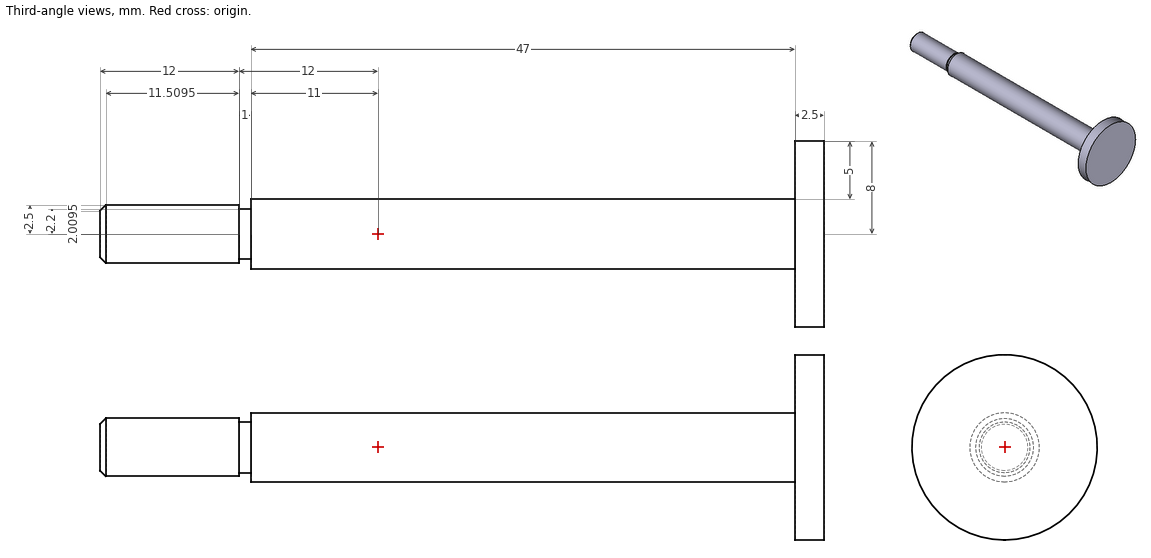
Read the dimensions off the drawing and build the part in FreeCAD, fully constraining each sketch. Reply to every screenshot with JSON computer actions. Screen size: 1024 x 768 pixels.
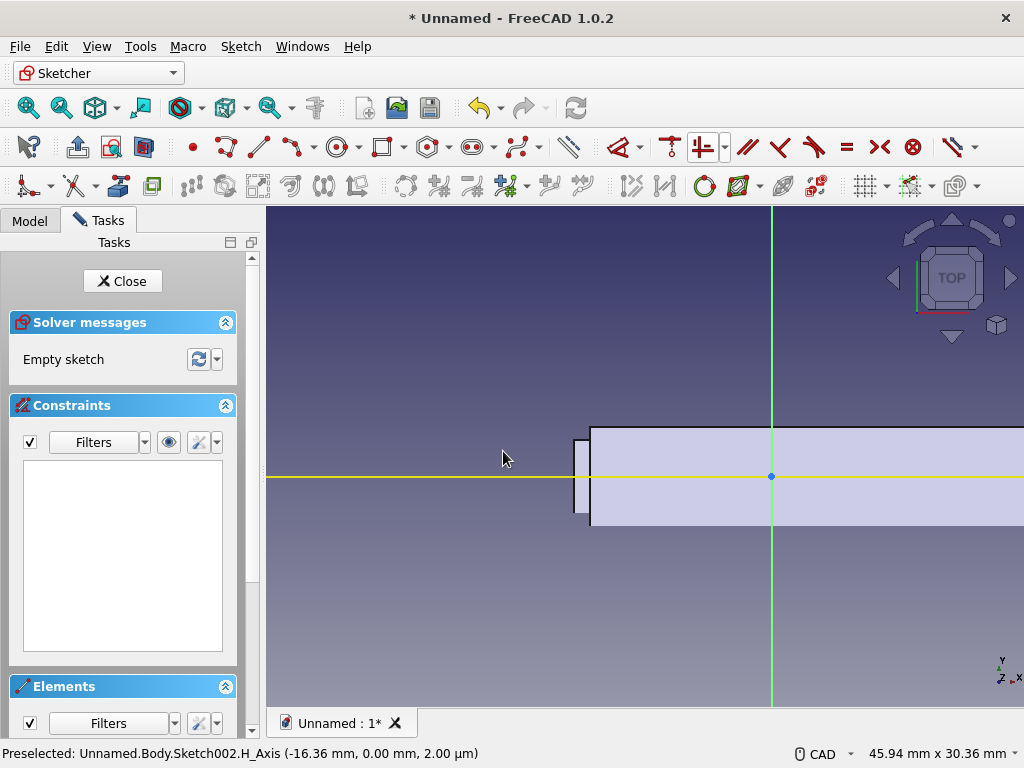
{"action": "key", "text": "g m"}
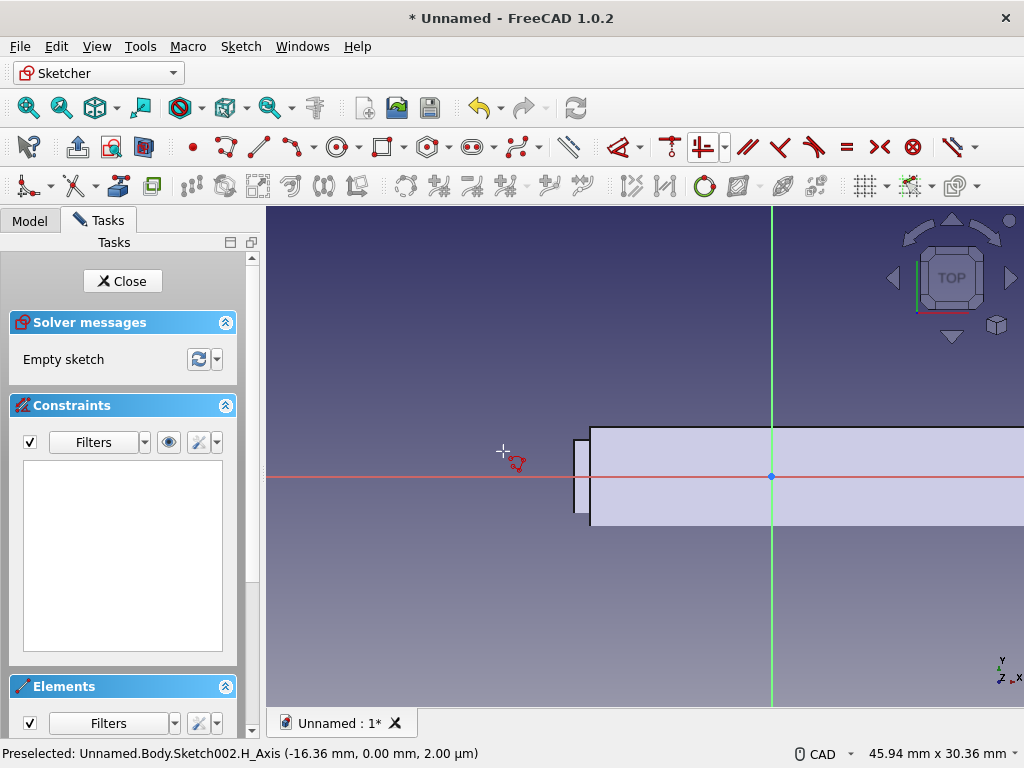
{"action": "left_click", "coordinate": [574, 477]}
{"action": "left_click", "coordinate": [574, 435]}
{"action": "left_click", "coordinate": [384, 435]}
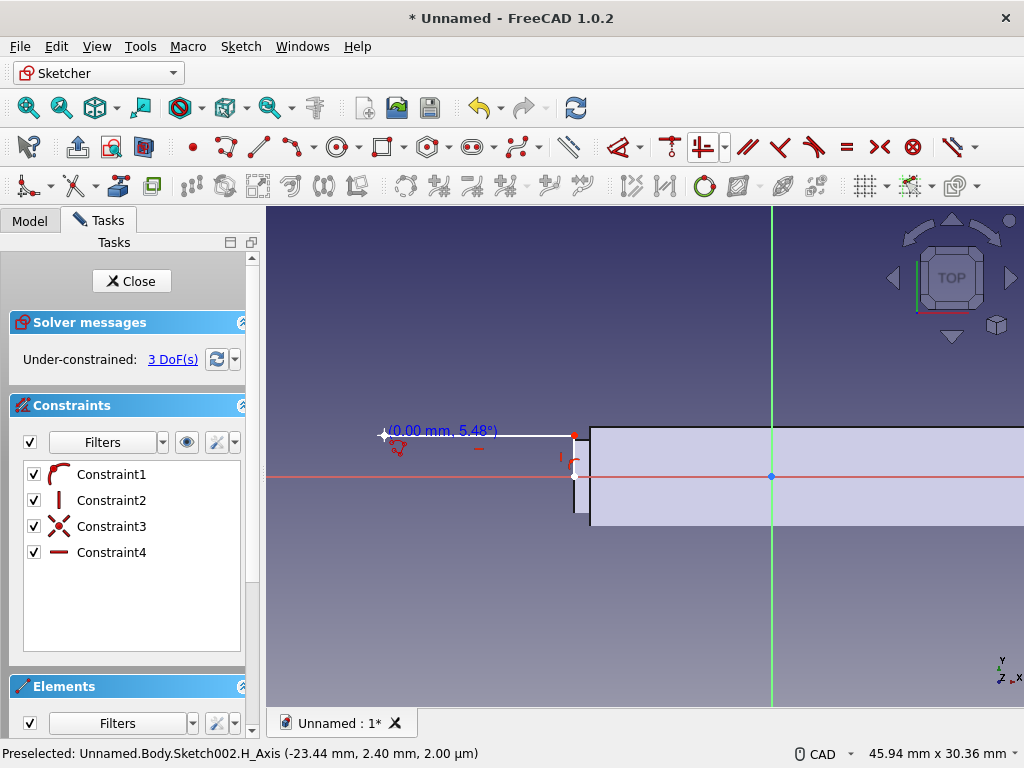
{"action": "scroll", "coordinate": [376, 443], "scroll_direction": "up", "scroll_amount": 2}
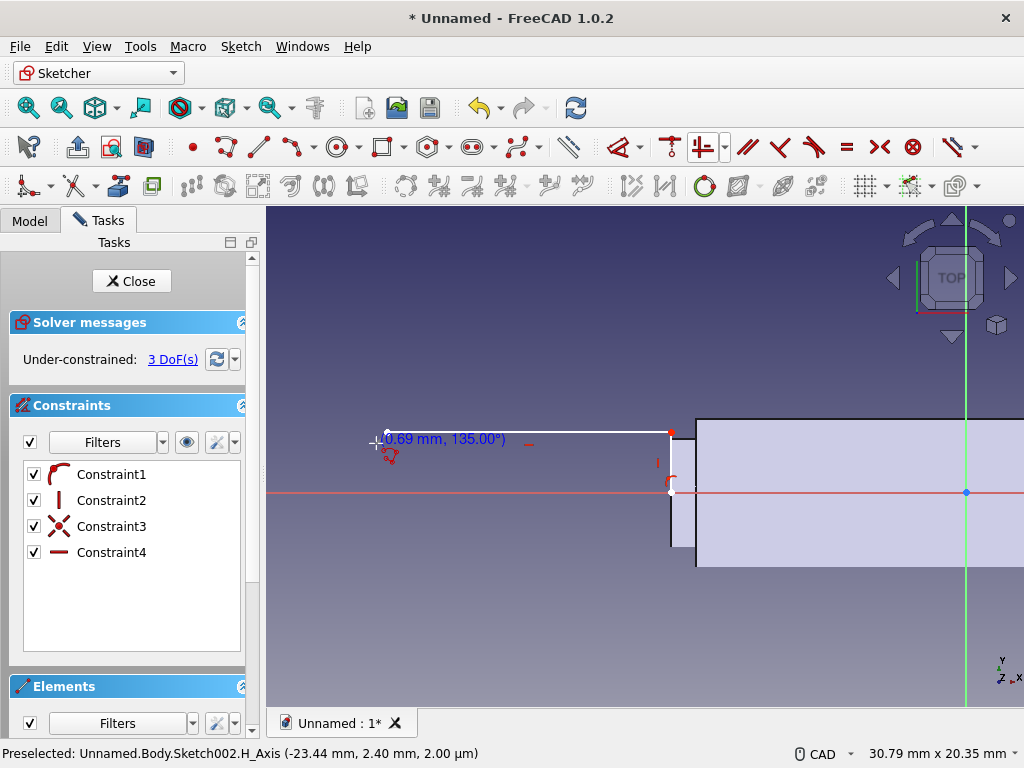
{"action": "left_click", "coordinate": [376, 443]}
{"action": "left_click", "coordinate": [376, 484]}
{"action": "left_click", "coordinate": [671, 493]}
{"action": "key", "text": "Escape"}
{"action": "key", "text": "Escape"}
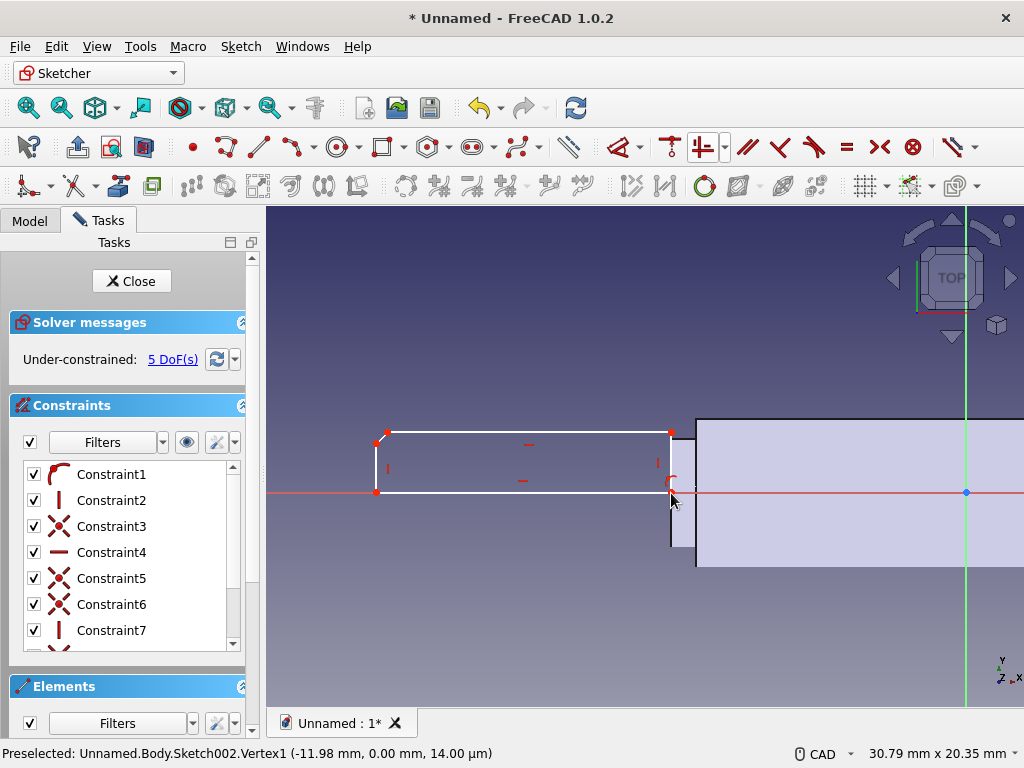
{"action": "left_click", "coordinate": [618, 148]}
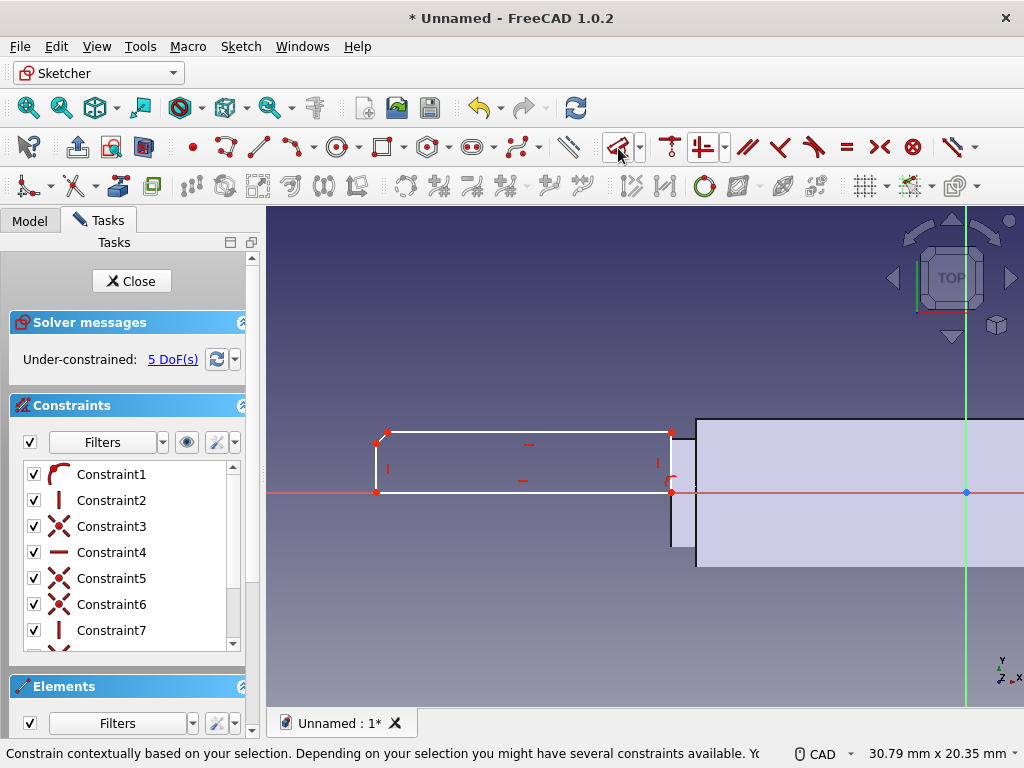
{"action": "left_click", "coordinate": [465, 493]}
{"action": "left_click", "coordinate": [524, 527]}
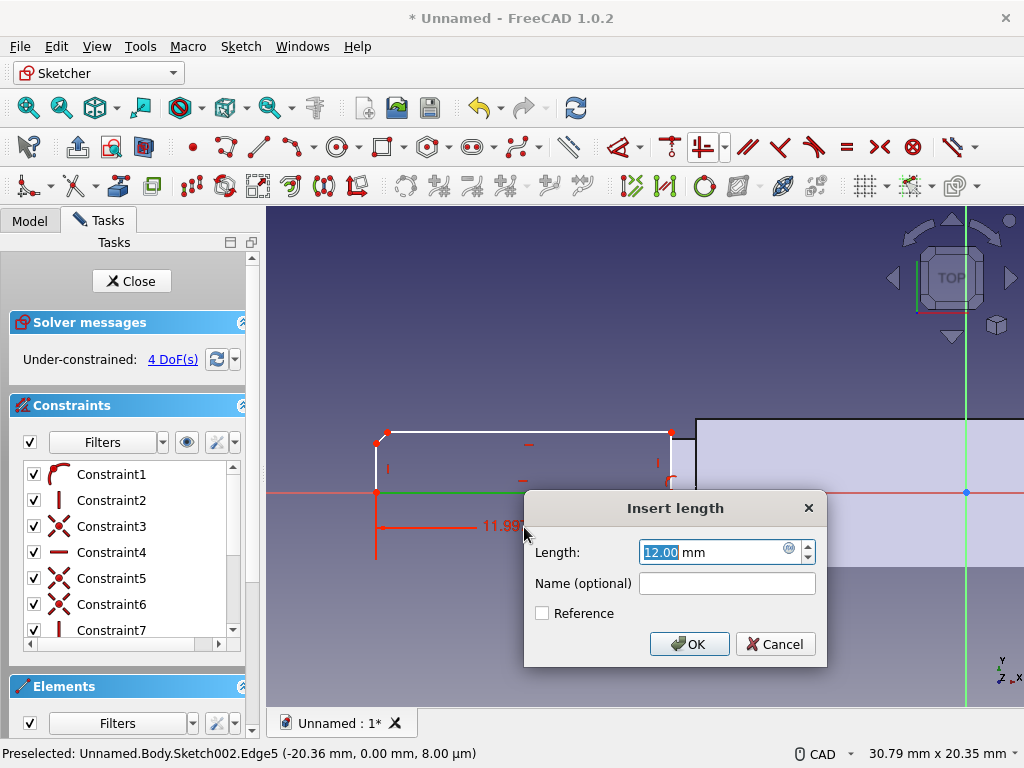
{"action": "type", "text": "12"}
{"action": "key", "text": "Return"}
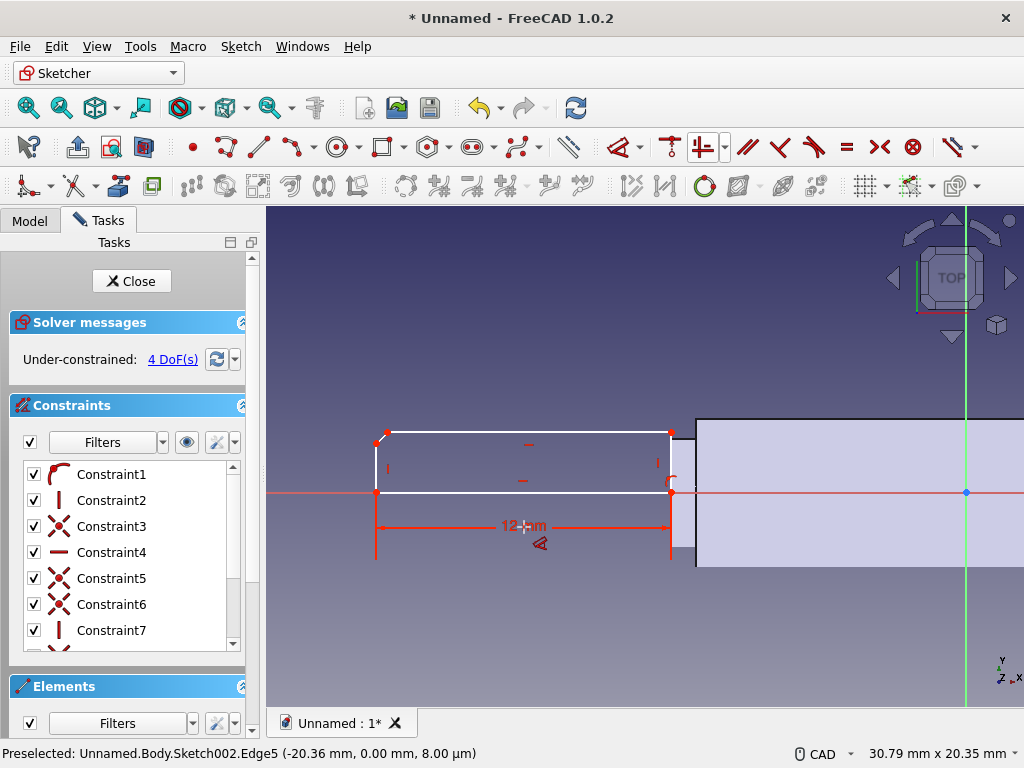
{"action": "left_click", "coordinate": [671, 475]}
{"action": "left_click", "coordinate": [705, 463]}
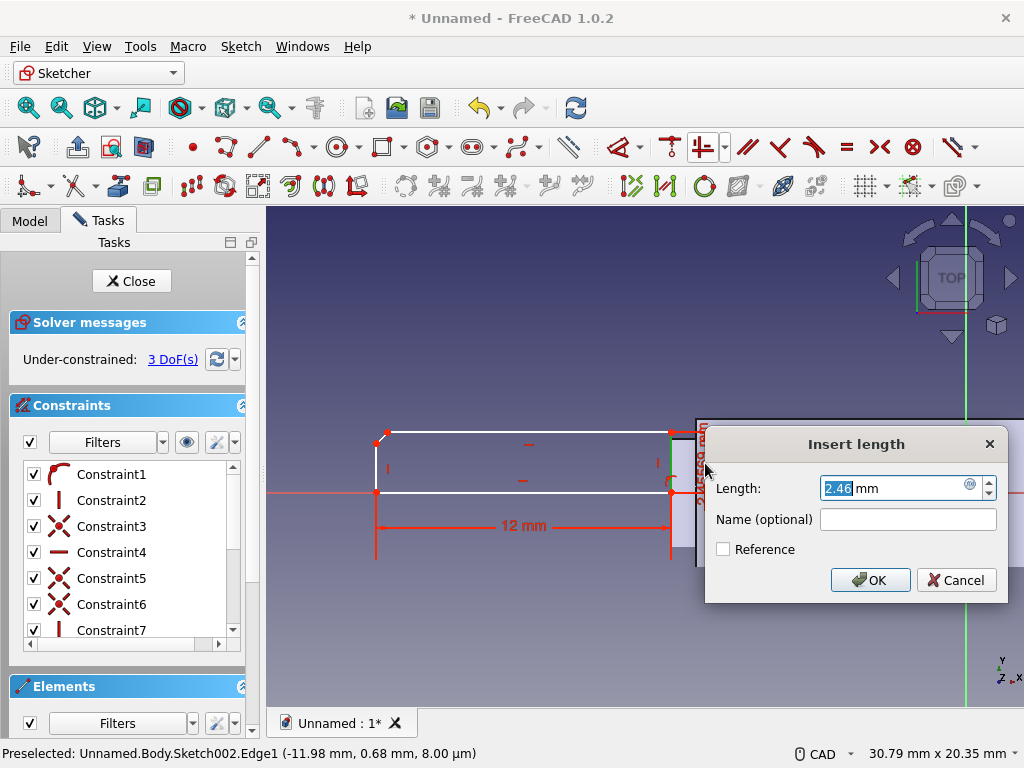
{"action": "type", "text": "2.5"}
{"action": "key", "text": "Return"}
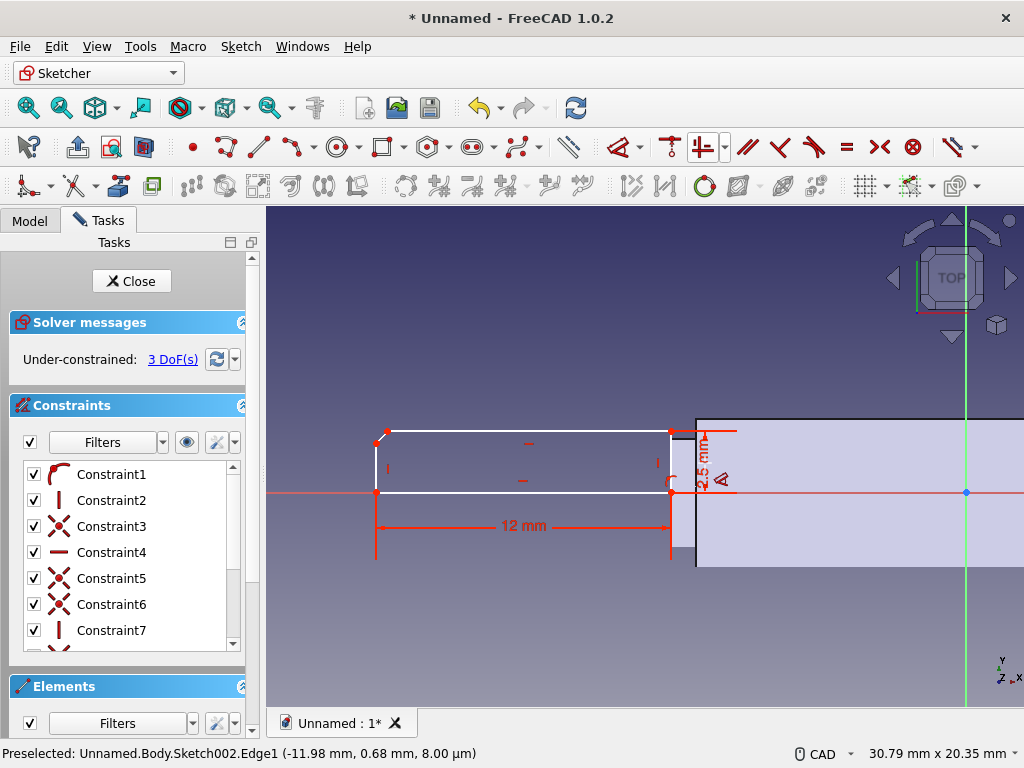
{"action": "left_click", "coordinate": [671, 493]}
{"action": "left_click", "coordinate": [765, 527]}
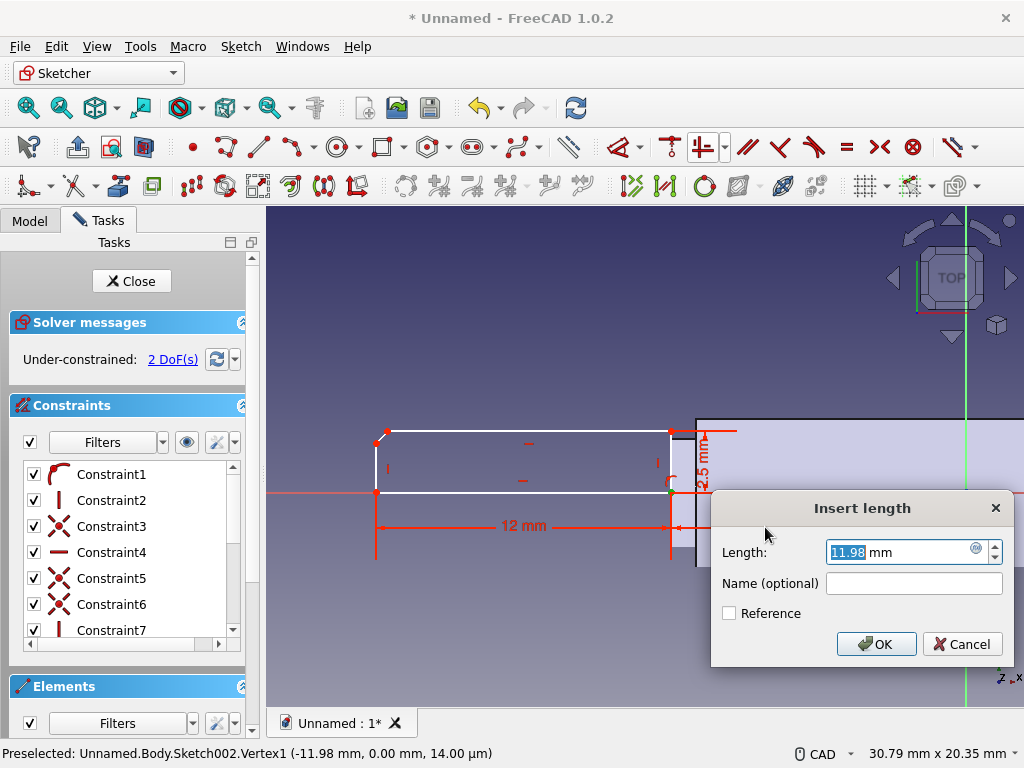
{"action": "type", "text": "12"}
{"action": "key", "text": "Return"}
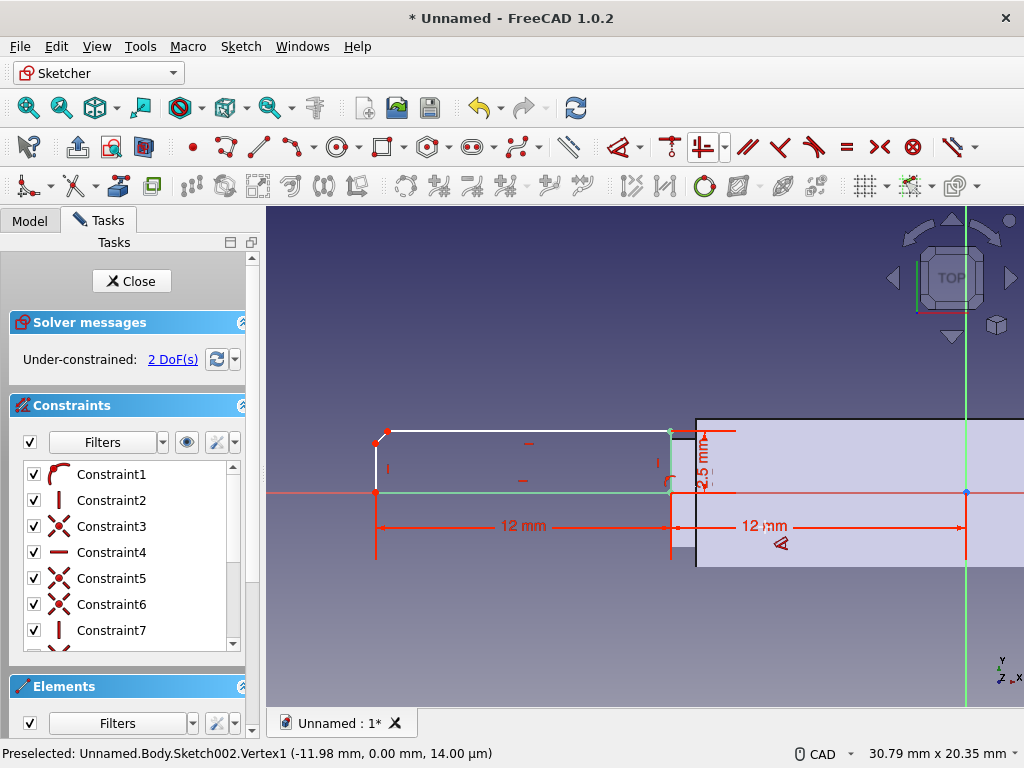
{"action": "left_click", "coordinate": [376, 459]}
{"action": "left_click", "coordinate": [342, 468]}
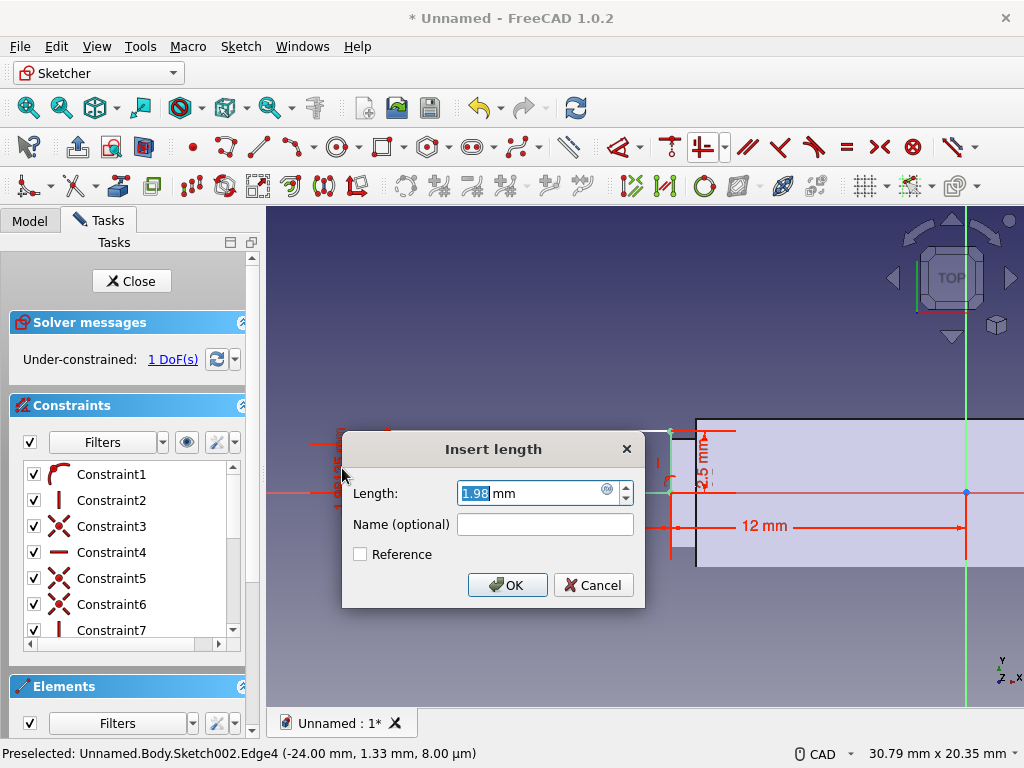
{"action": "type", "text": "2.0095"}
{"action": "key", "text": "Return"}